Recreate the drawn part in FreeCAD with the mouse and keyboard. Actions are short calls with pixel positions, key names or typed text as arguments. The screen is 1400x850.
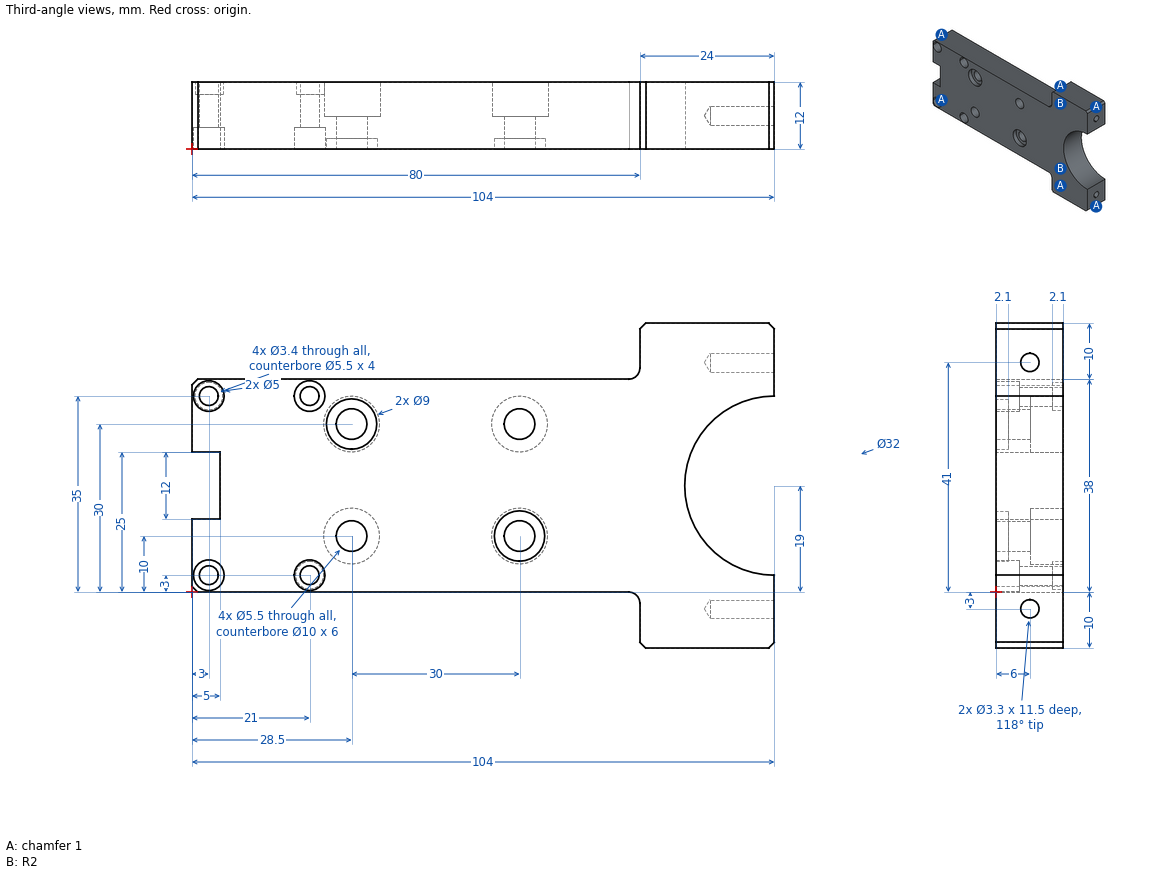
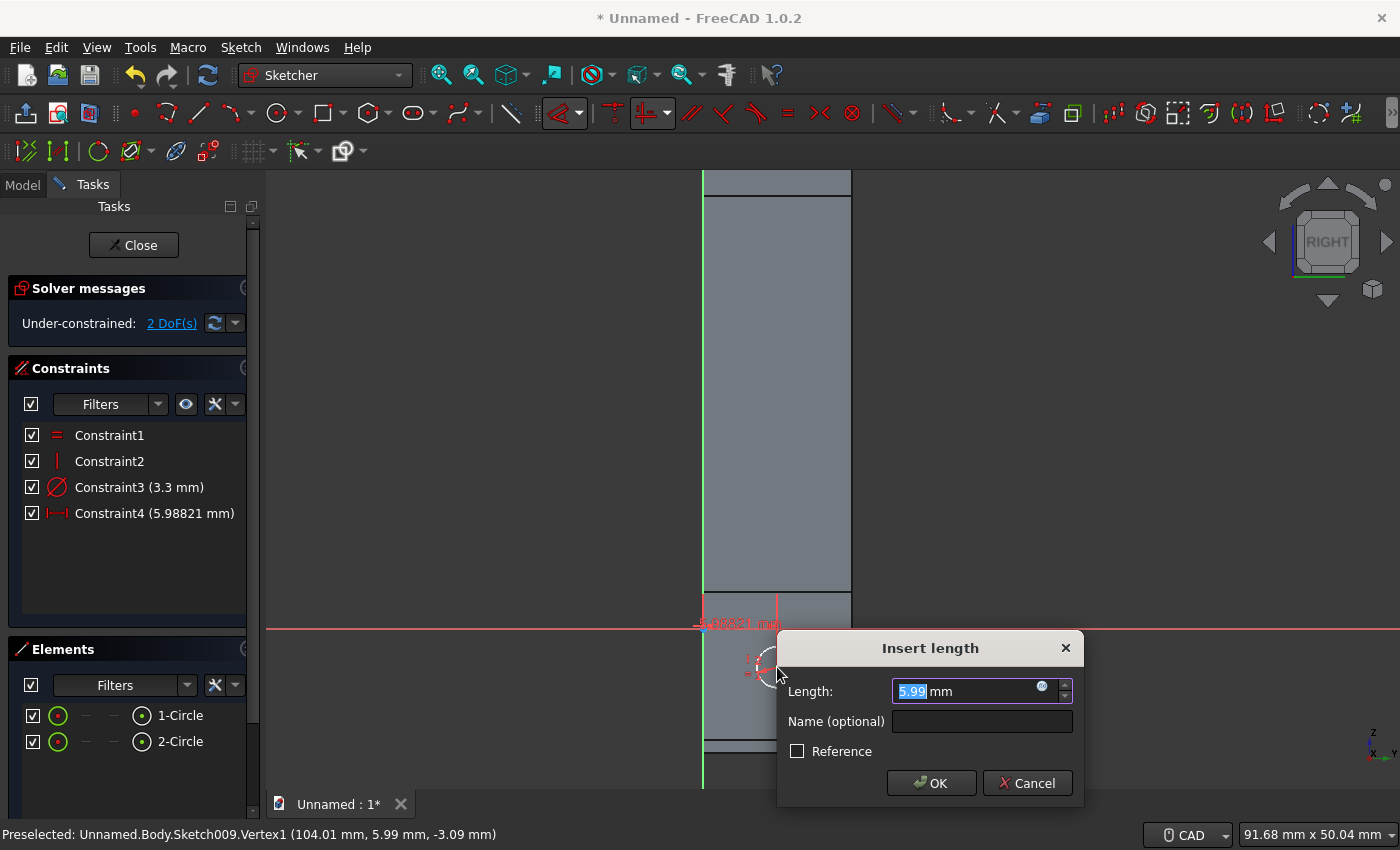
text(6)
key(Return)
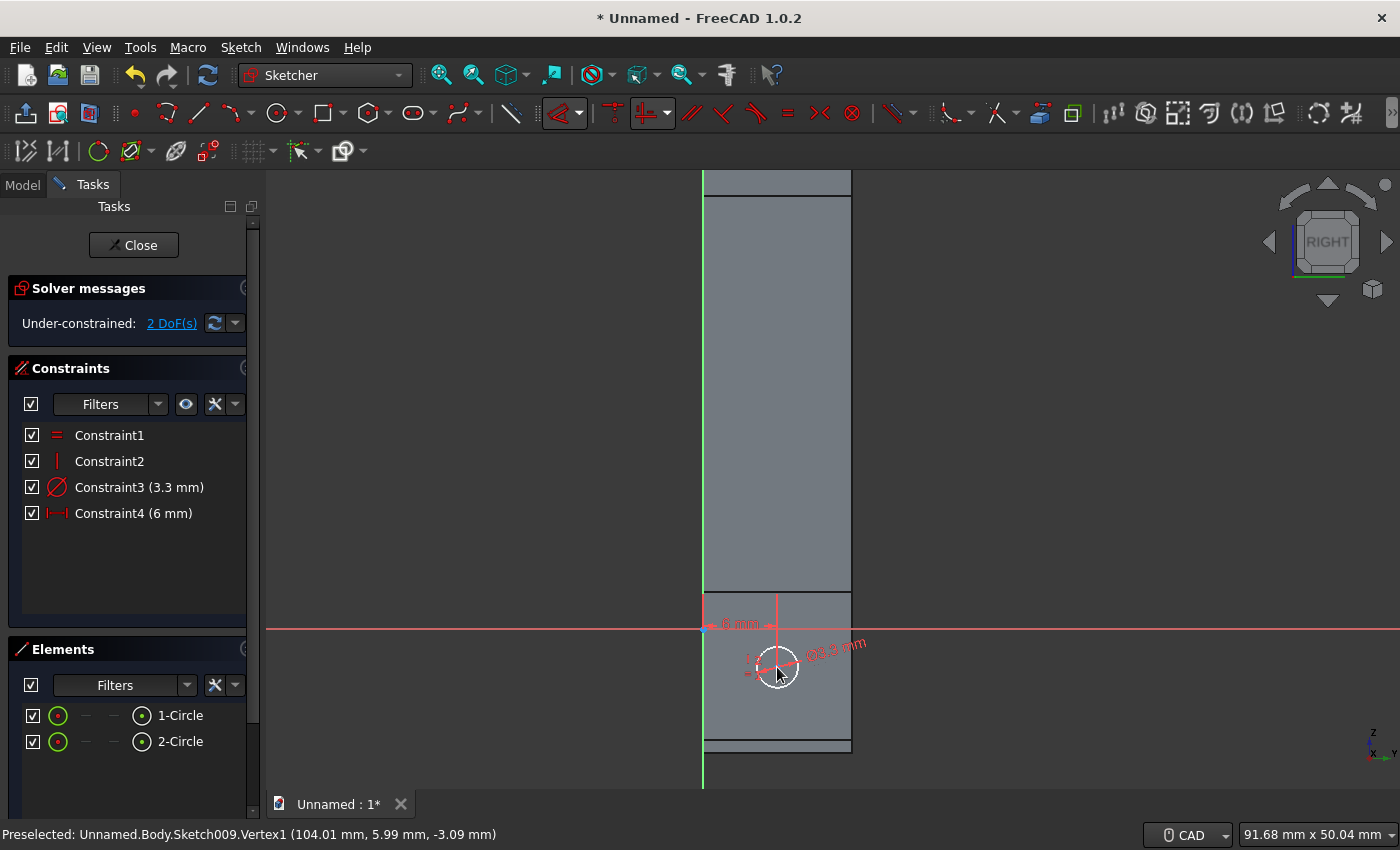
click(777, 667)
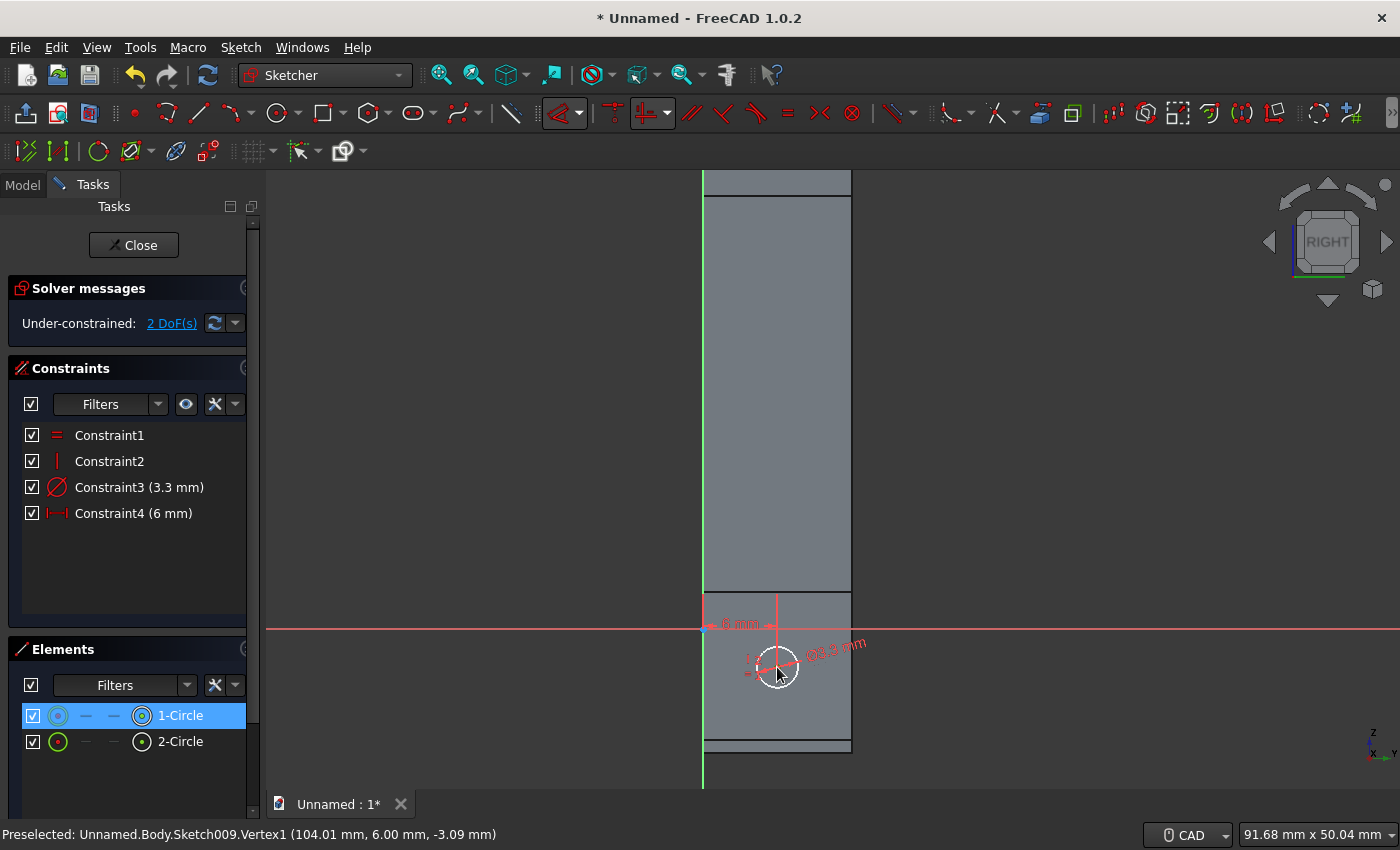
click(582, 114)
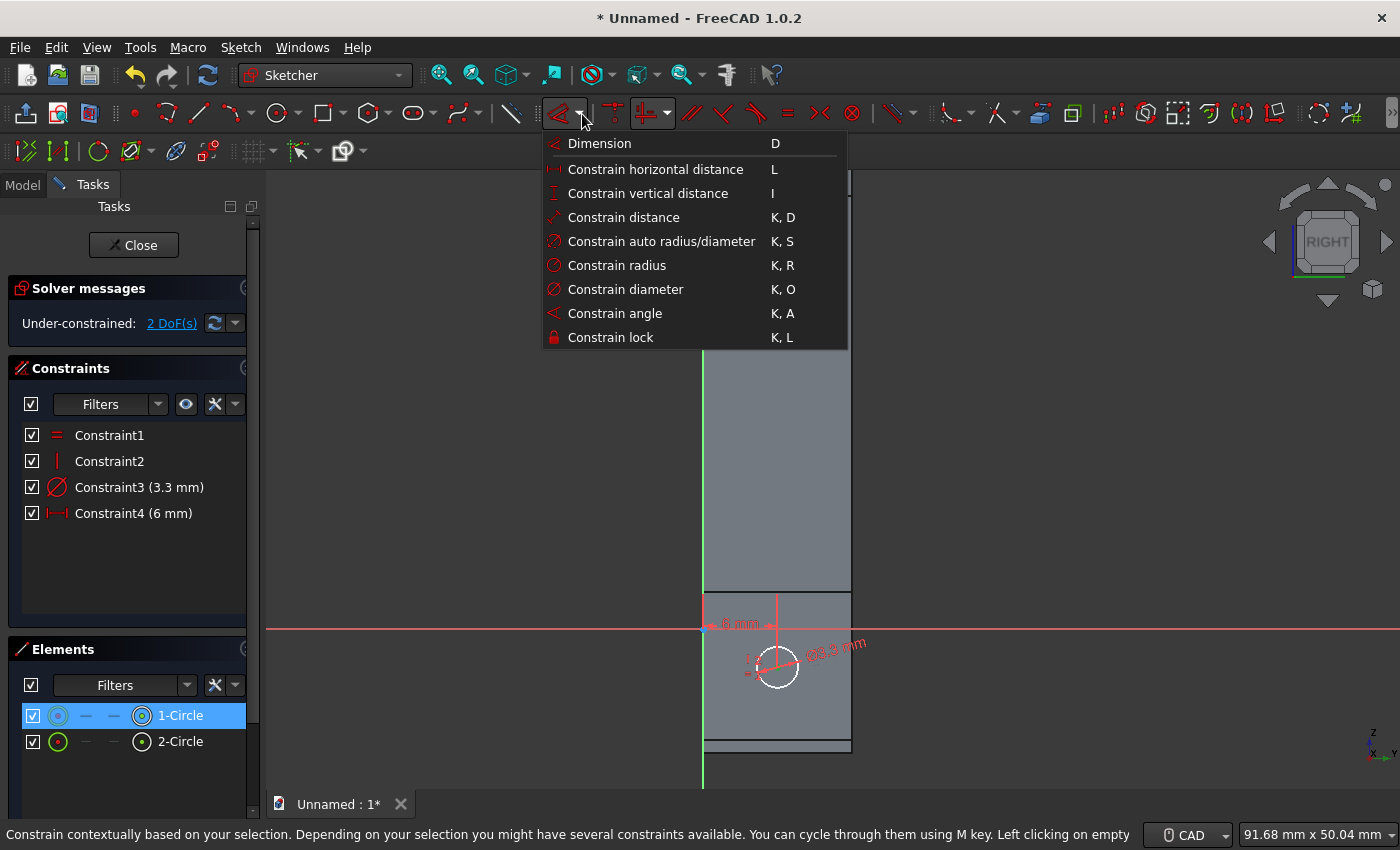
click(695, 193)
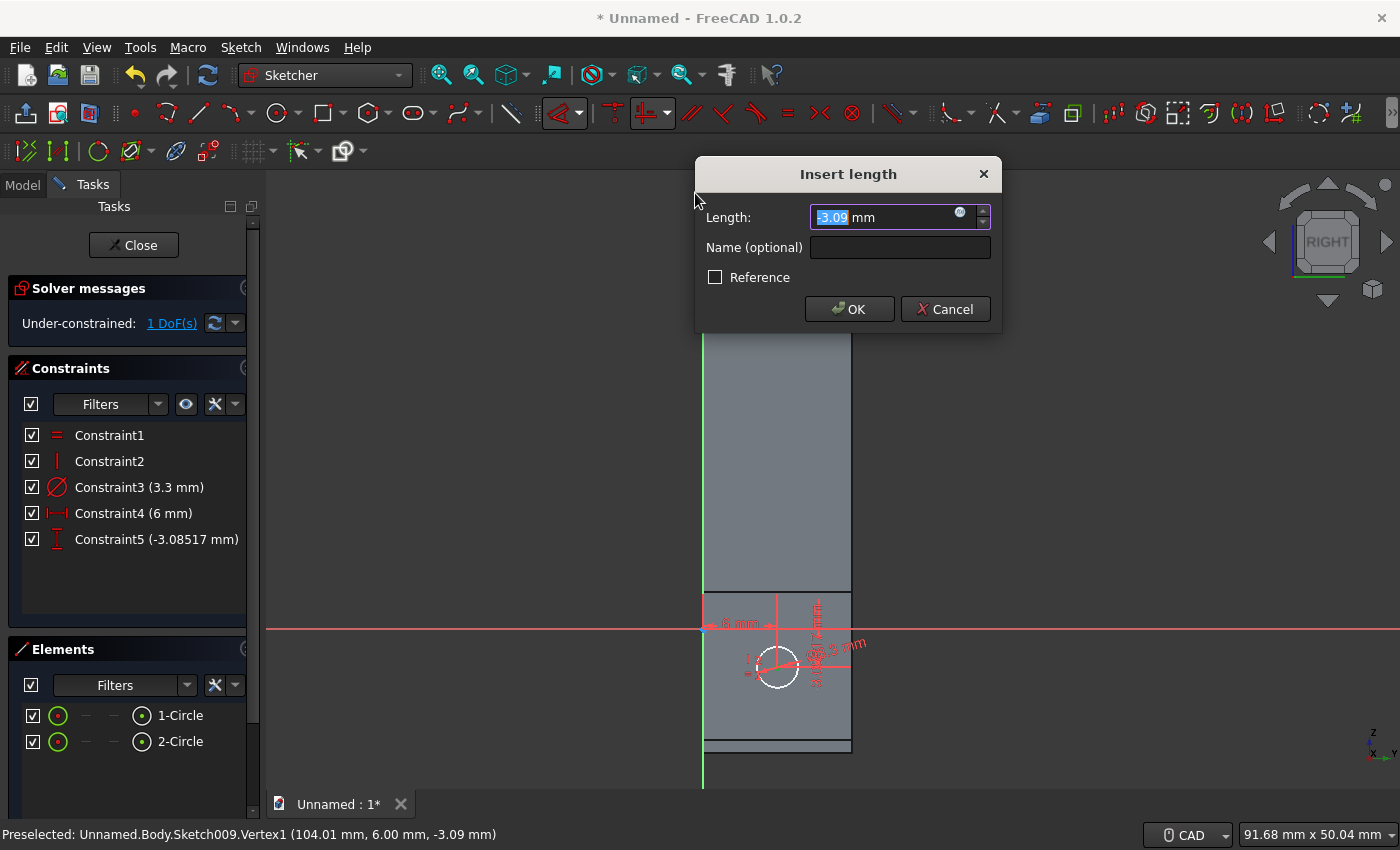
text(-3)
key(Return)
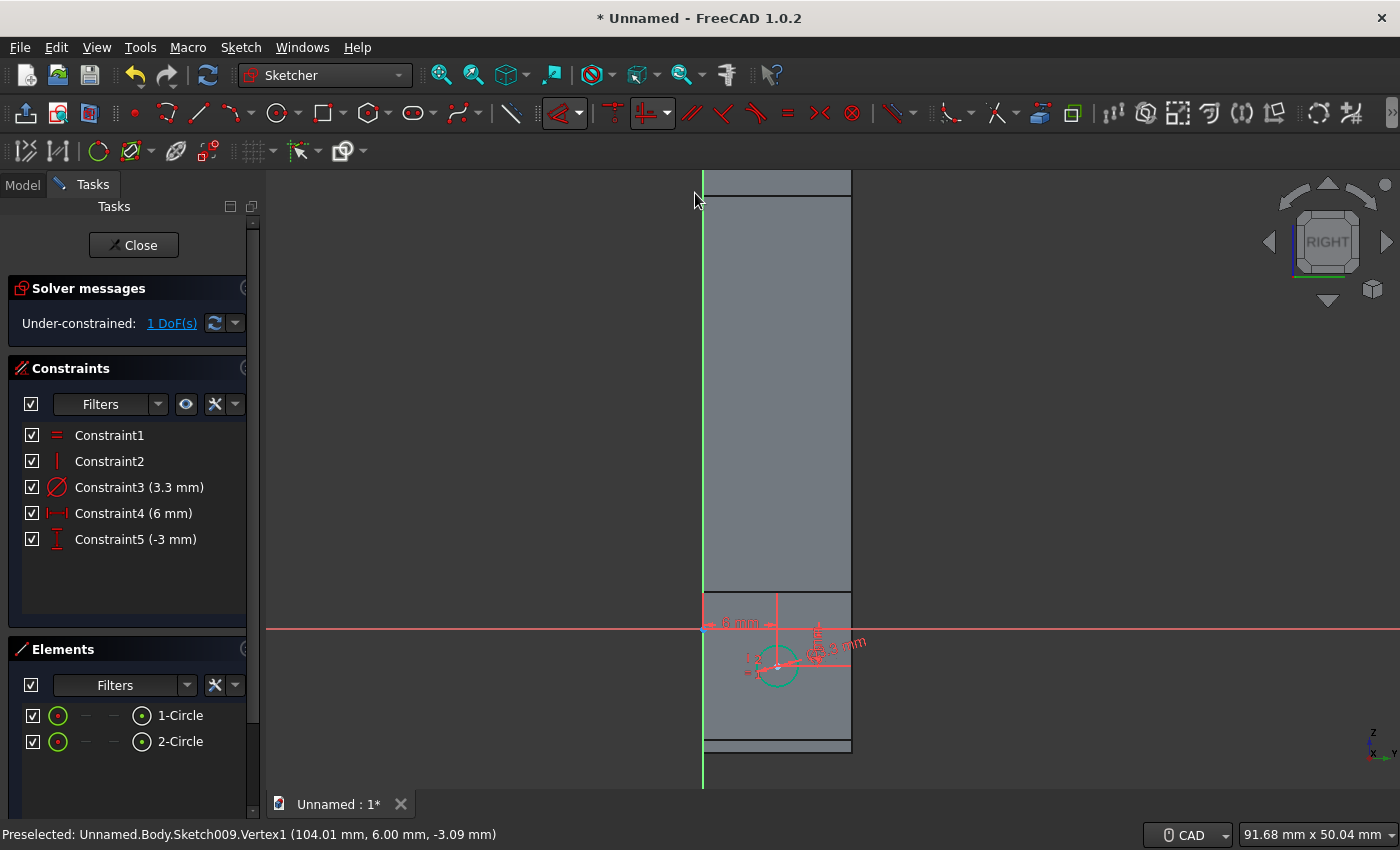
scroll(793, 653, down, 2)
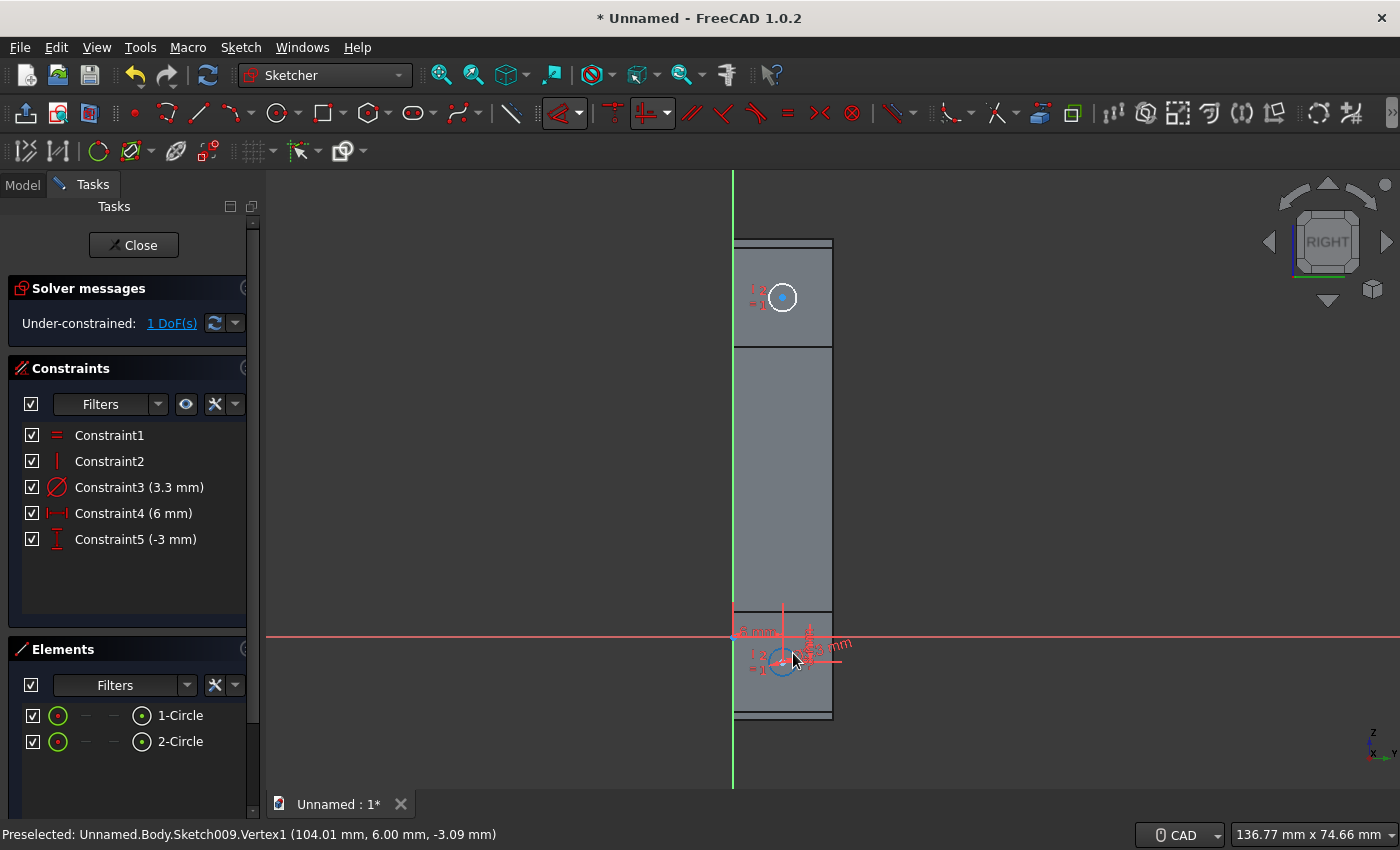
click(783, 298)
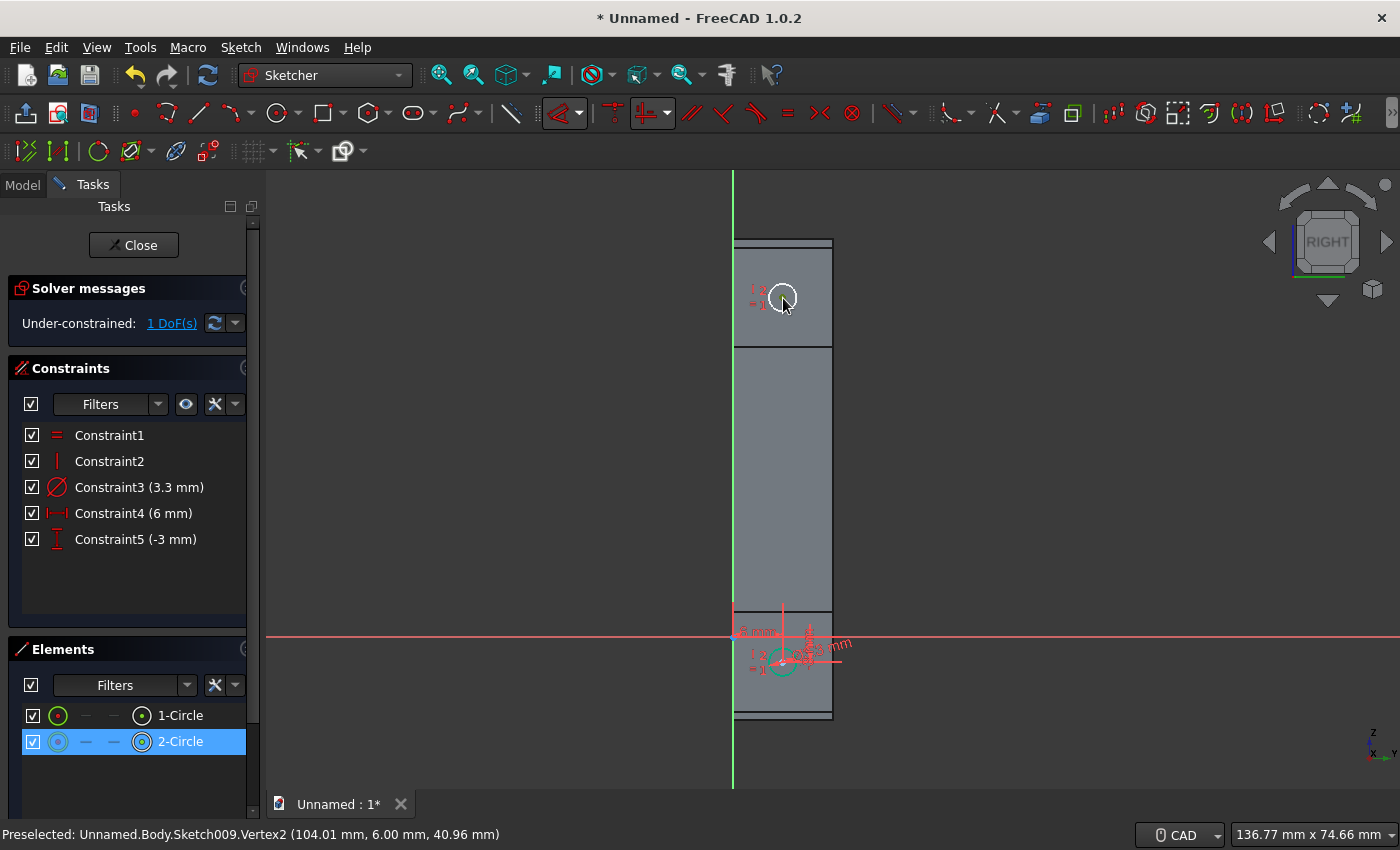
key(i)